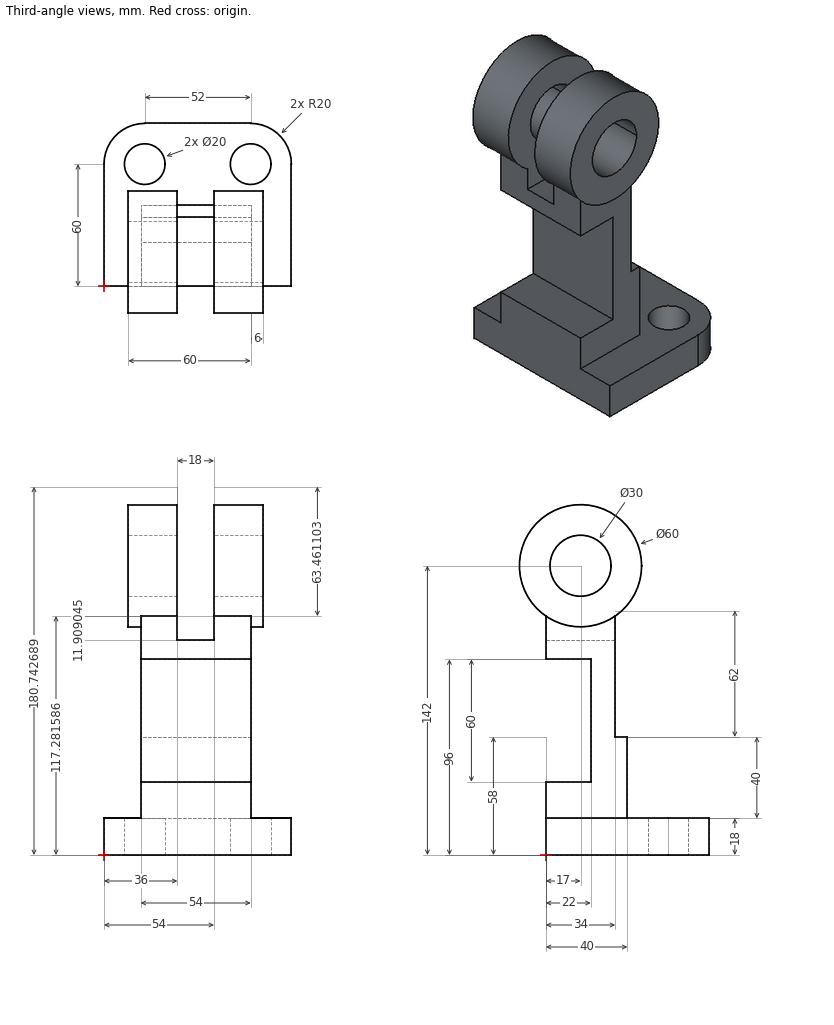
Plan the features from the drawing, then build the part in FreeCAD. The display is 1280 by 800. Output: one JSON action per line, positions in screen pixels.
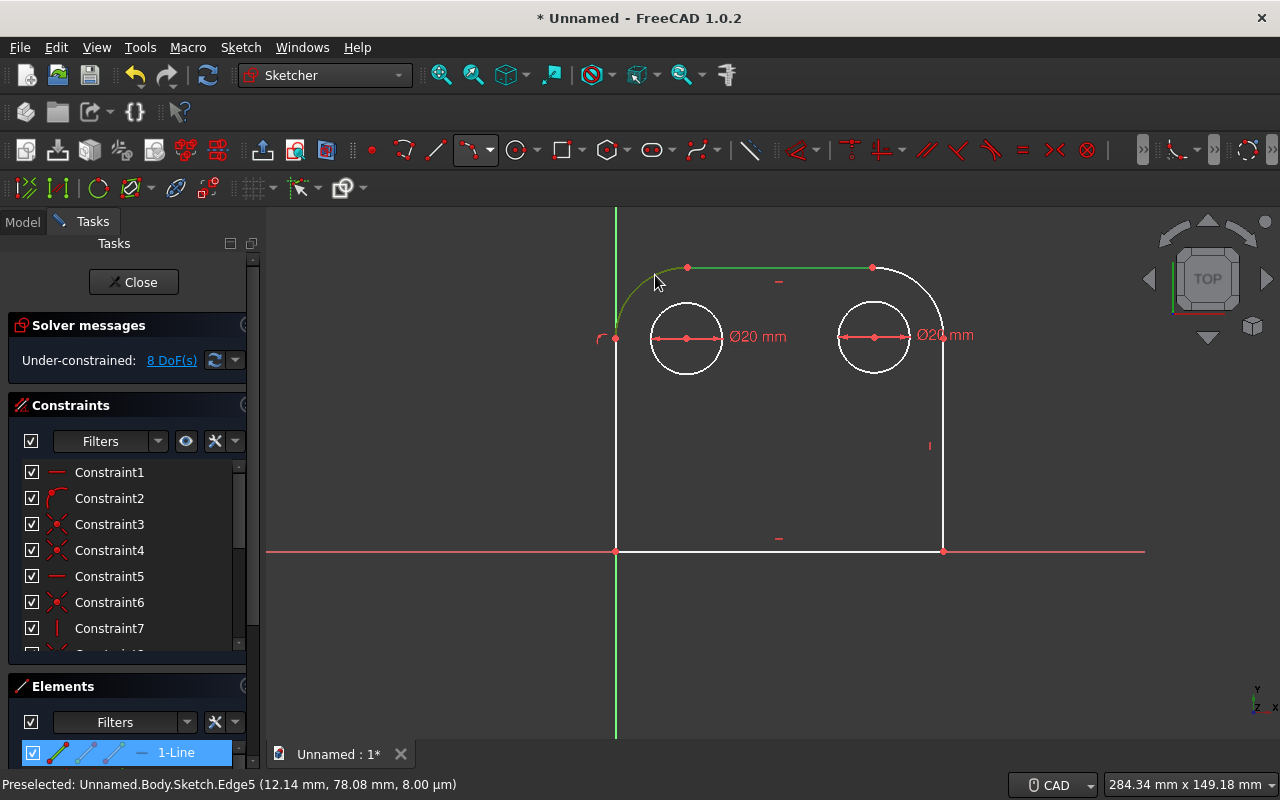
{"action": "left_click", "coordinate": [992, 150]}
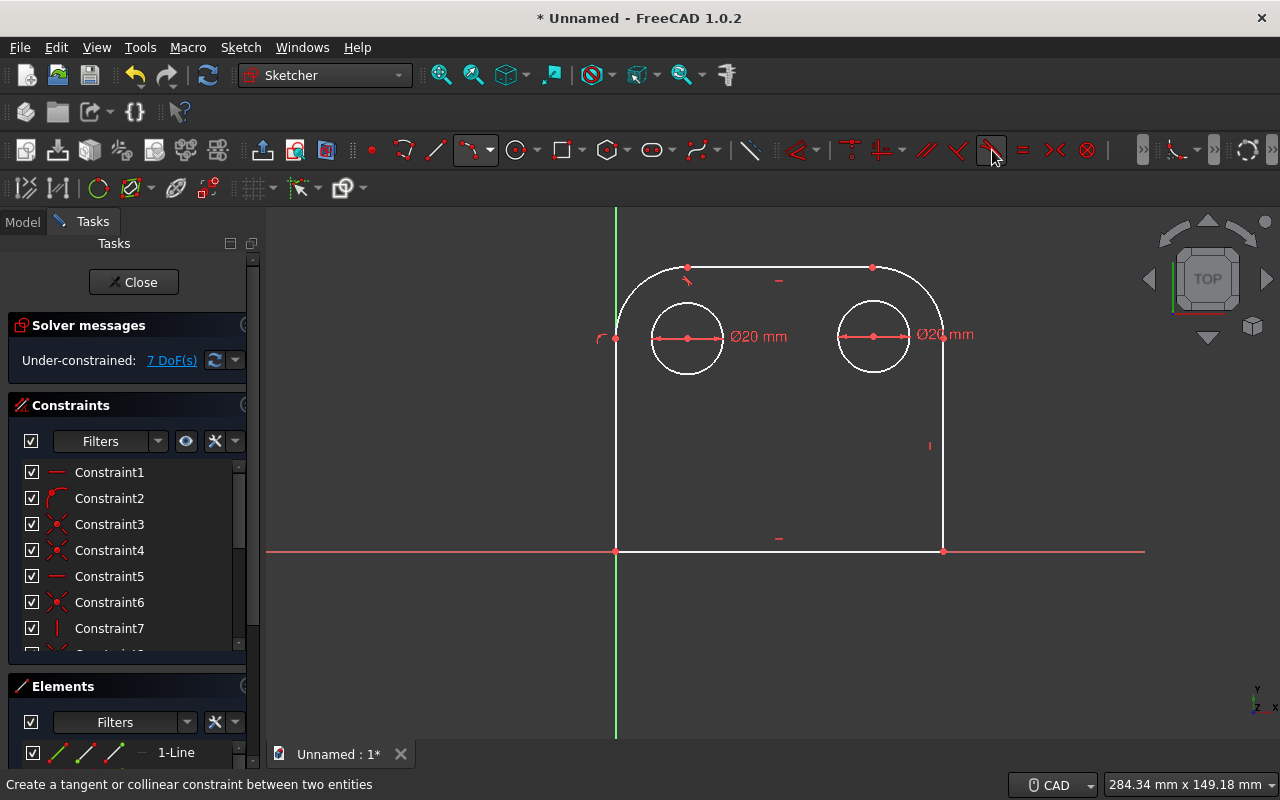
{"action": "left_click", "coordinate": [817, 267]}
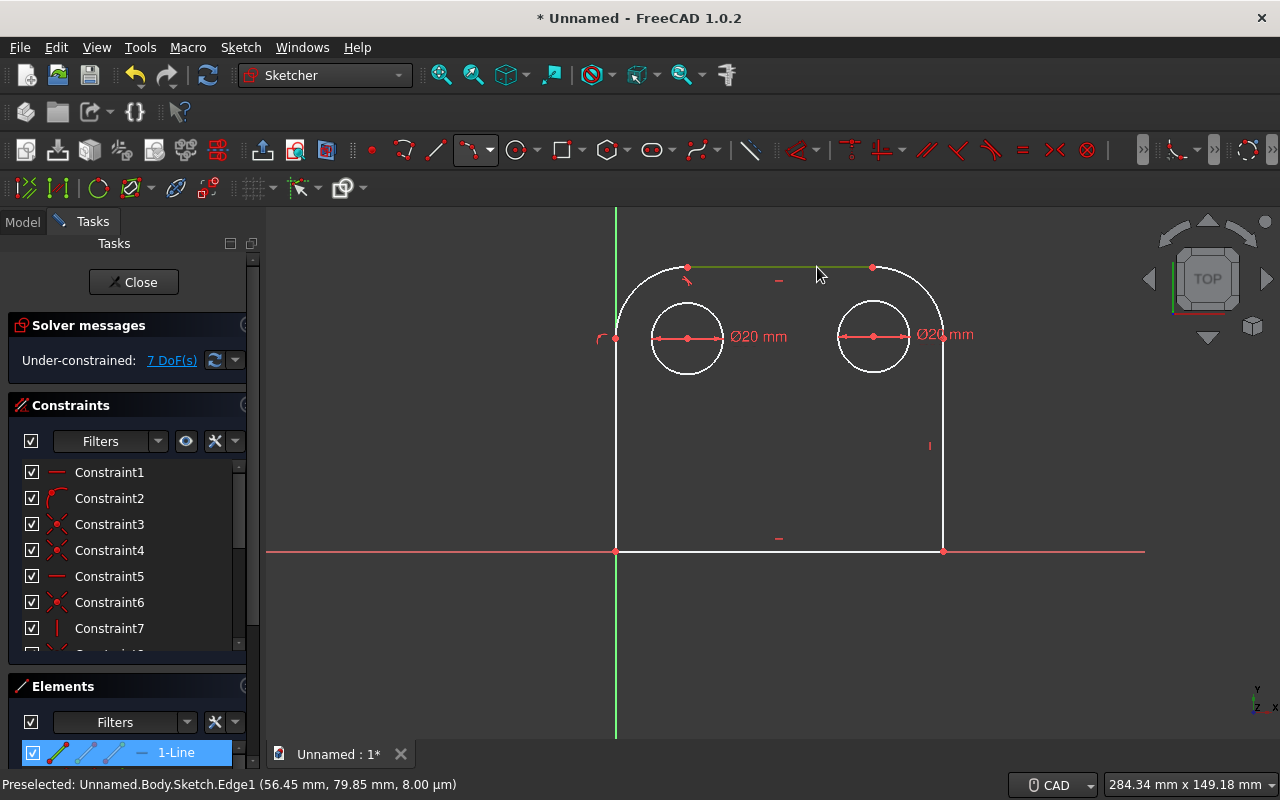
{"action": "left_click", "coordinate": [936, 306]}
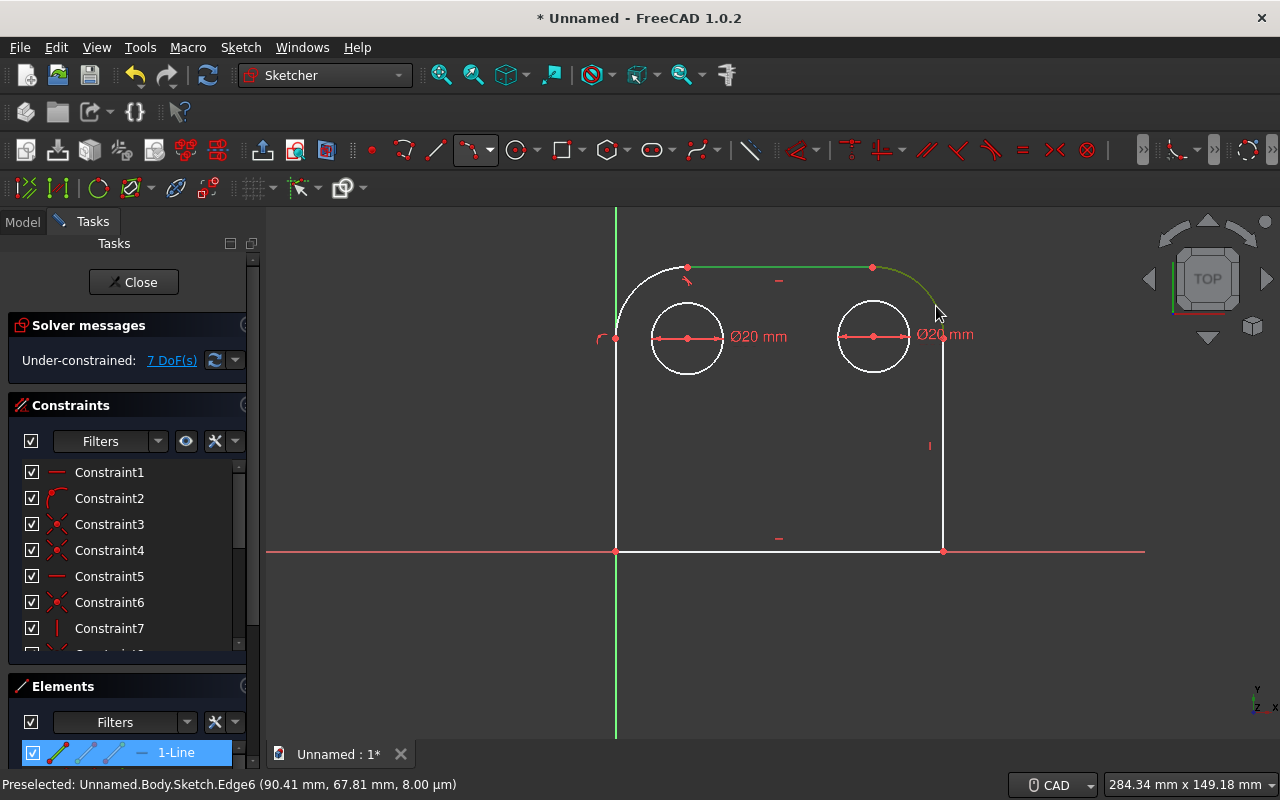
{"action": "left_click", "coordinate": [992, 150]}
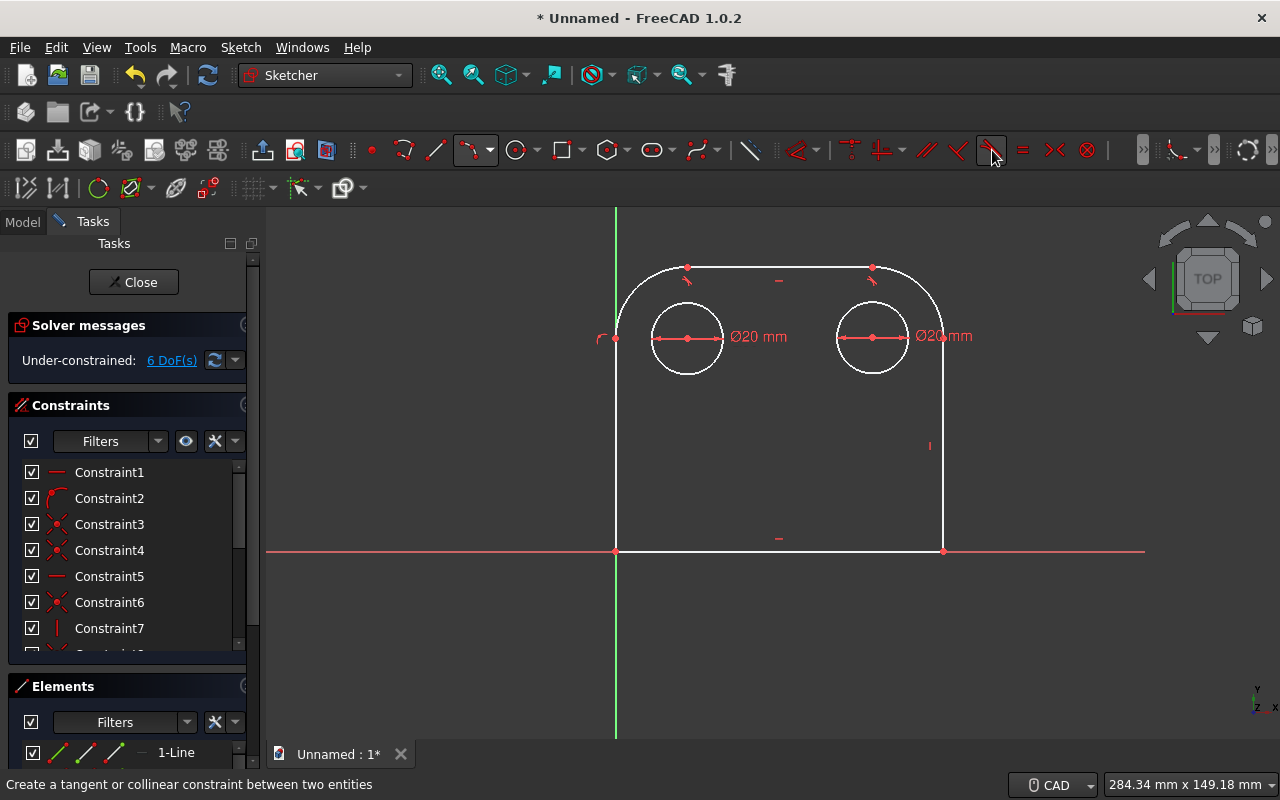
{"action": "left_click", "coordinate": [616, 402]}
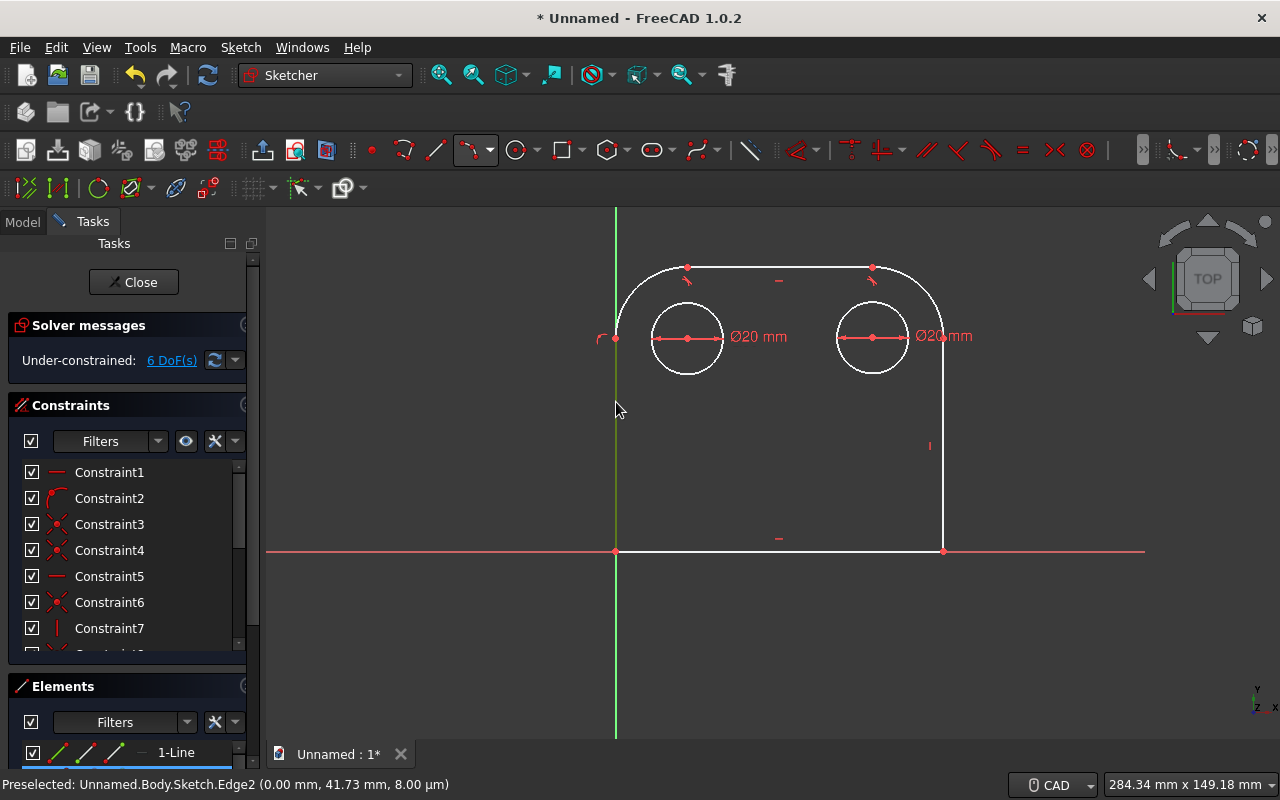
{"action": "left_click", "coordinate": [655, 275]}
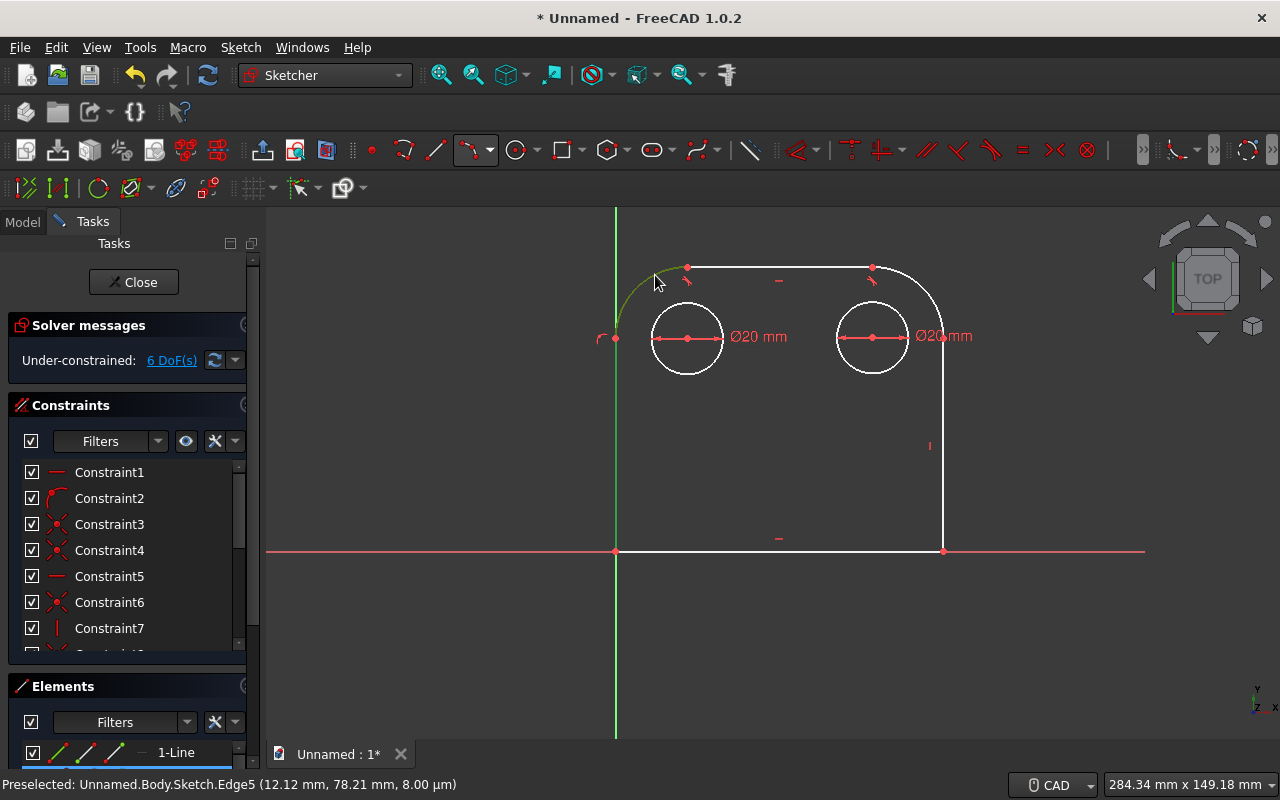
{"action": "left_click", "coordinate": [992, 150]}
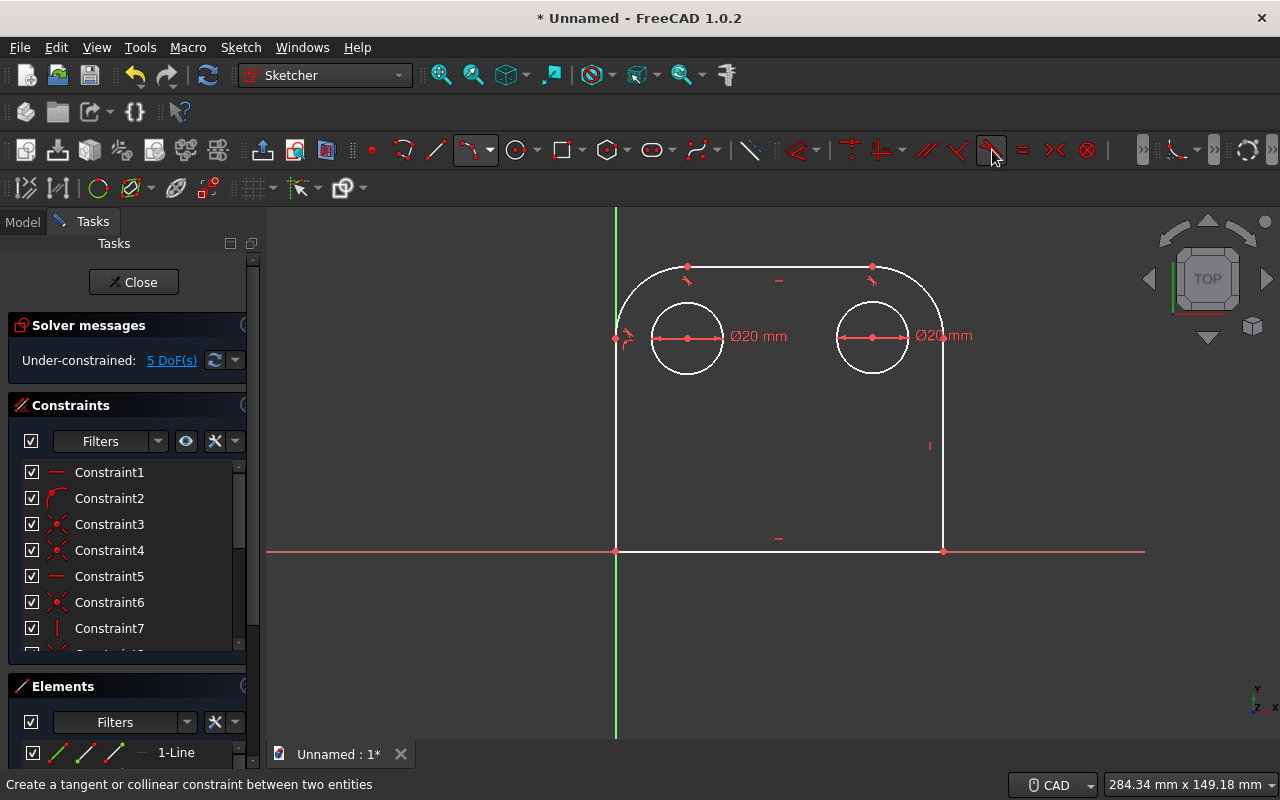
{"action": "left_click", "coordinate": [943, 488]}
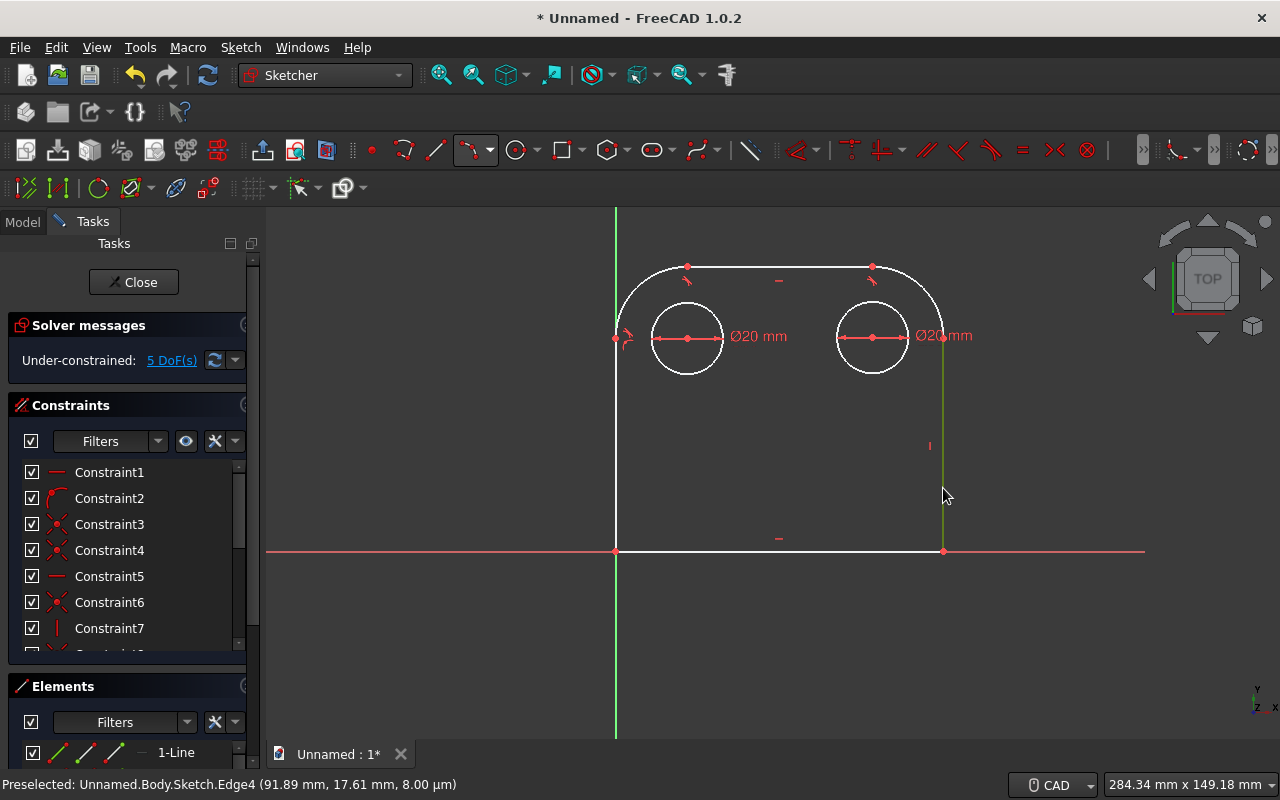
{"action": "left_click", "coordinate": [936, 306]}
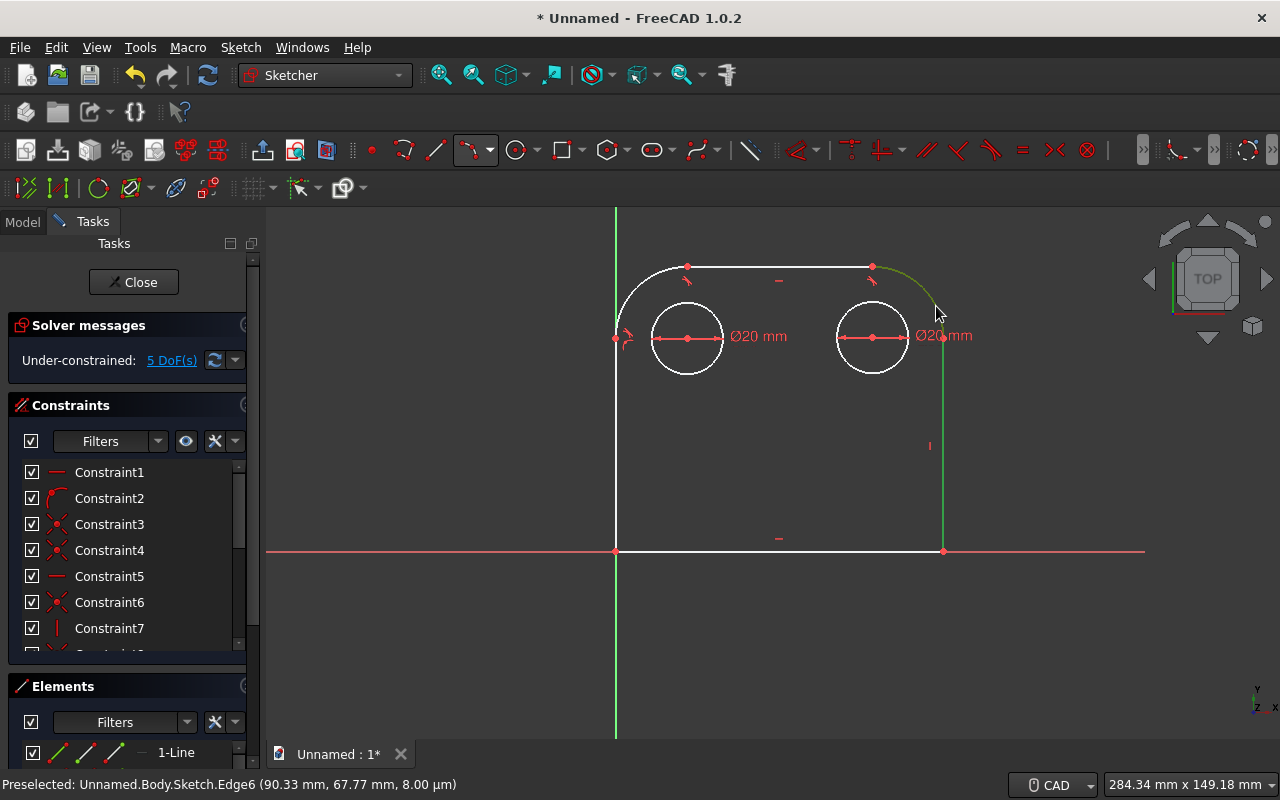
{"action": "left_click", "coordinate": [992, 150]}